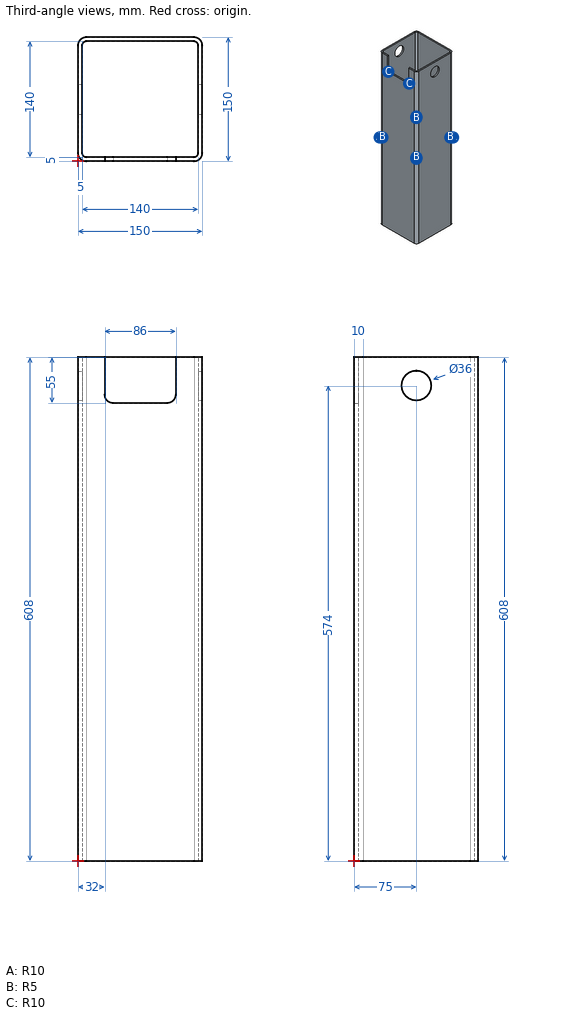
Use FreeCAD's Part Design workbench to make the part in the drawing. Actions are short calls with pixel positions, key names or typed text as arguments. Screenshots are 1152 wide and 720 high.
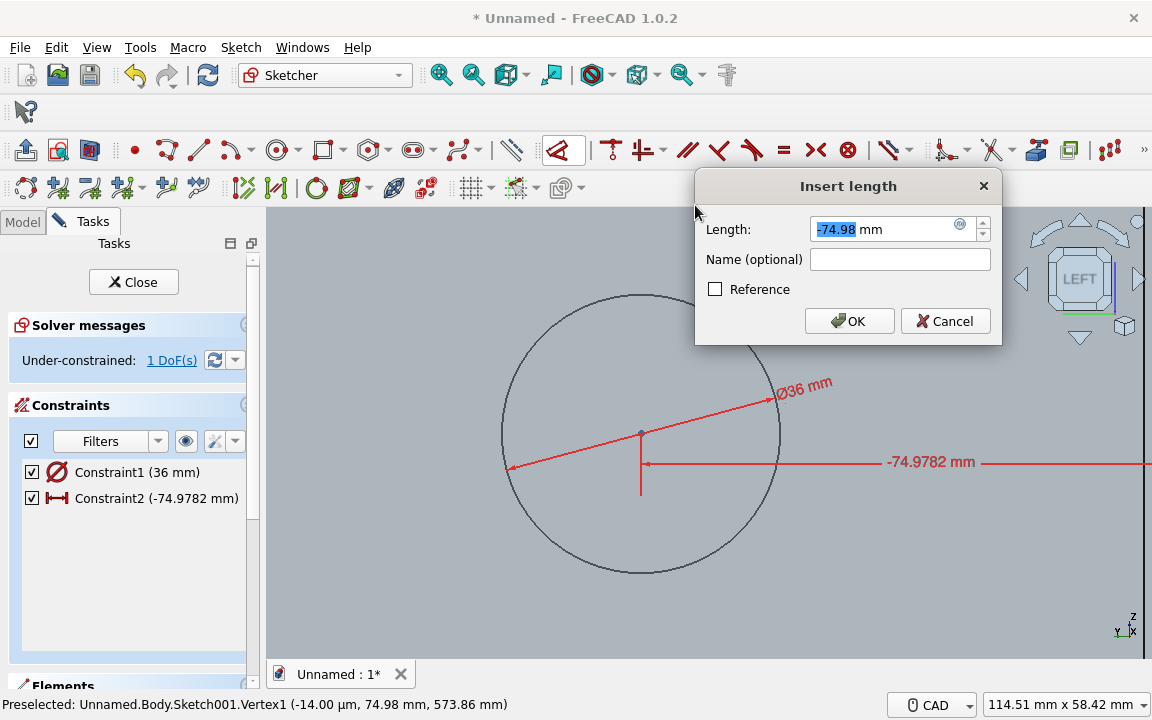
text(-75)
key(Return)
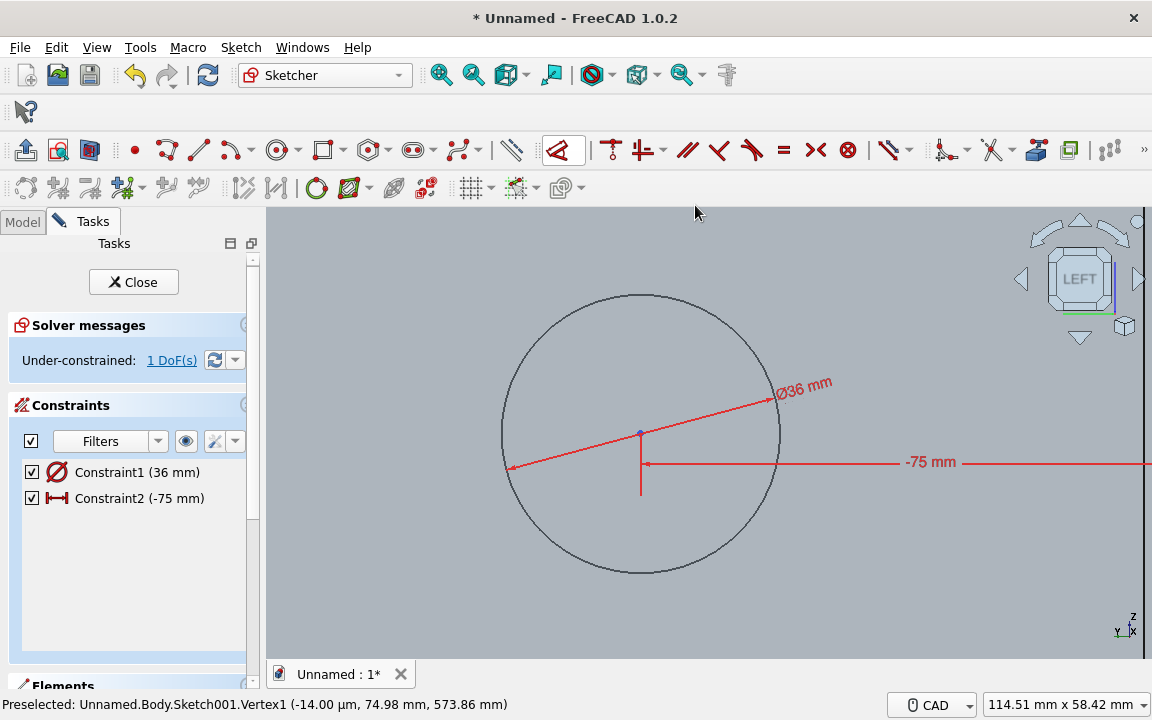
click(641, 434)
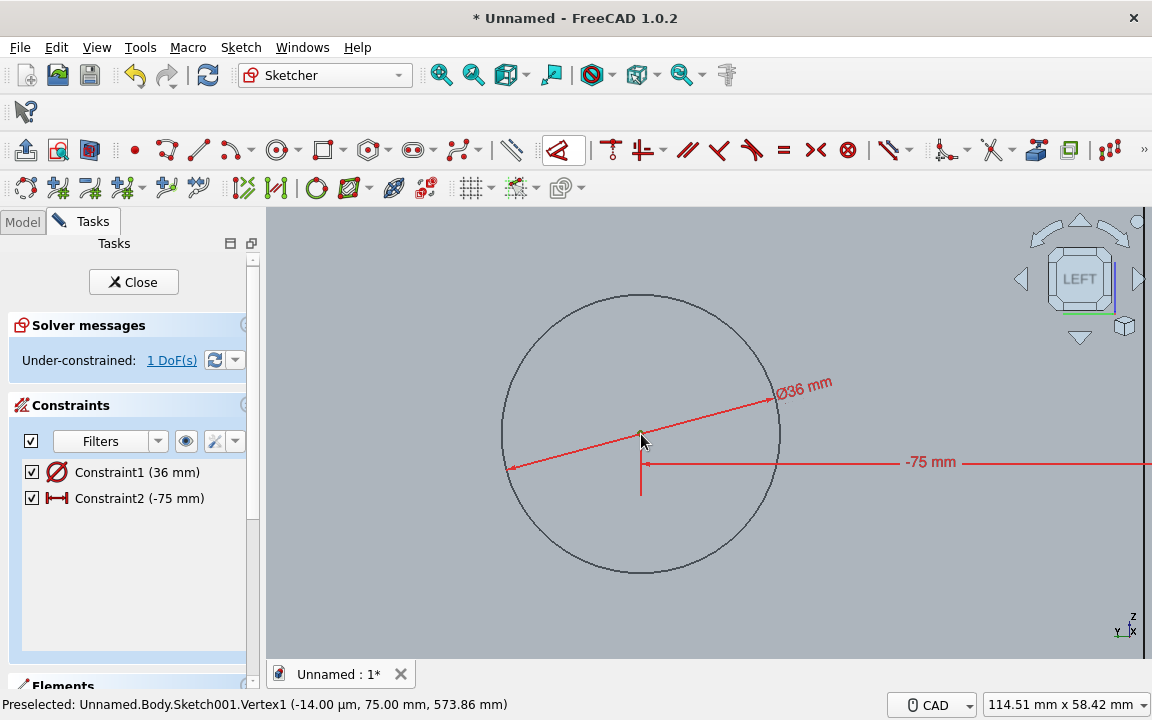
key(i)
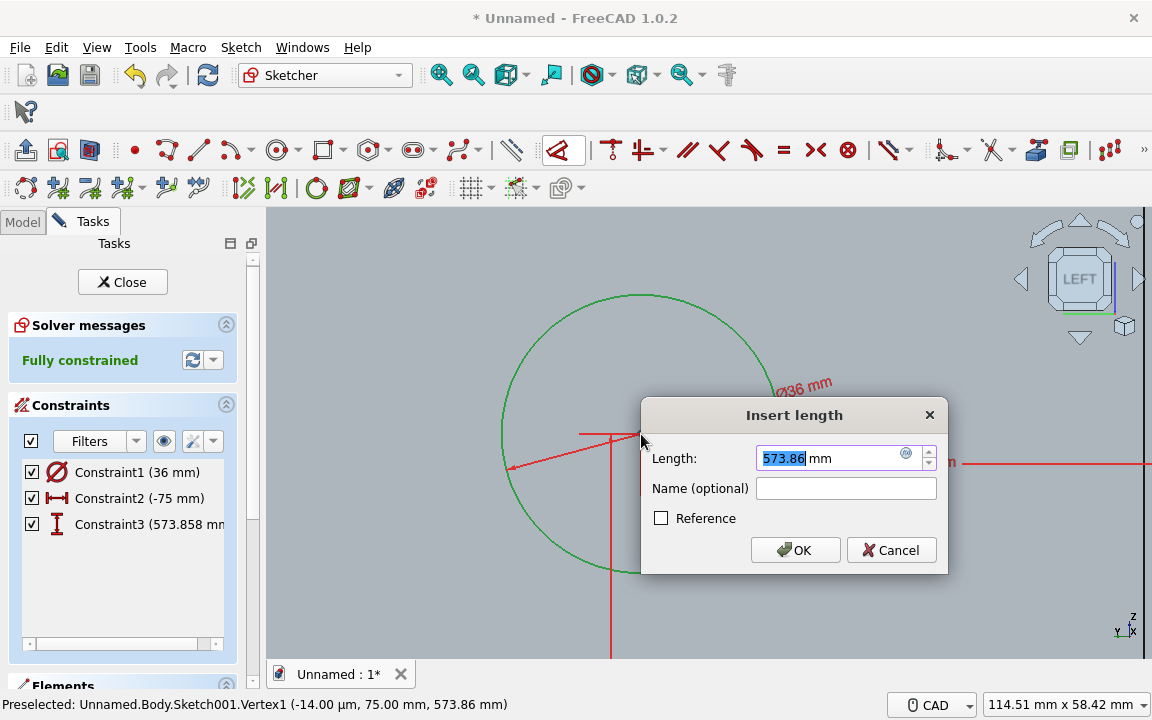
text(574)
key(Return)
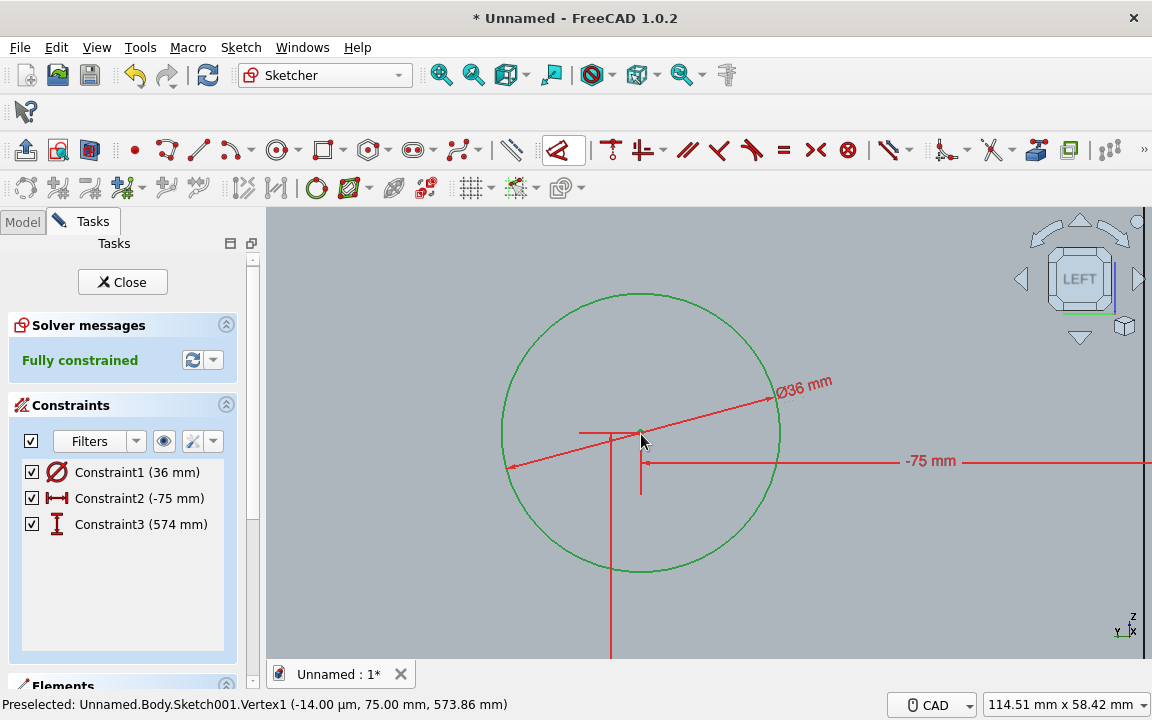
click(123, 282)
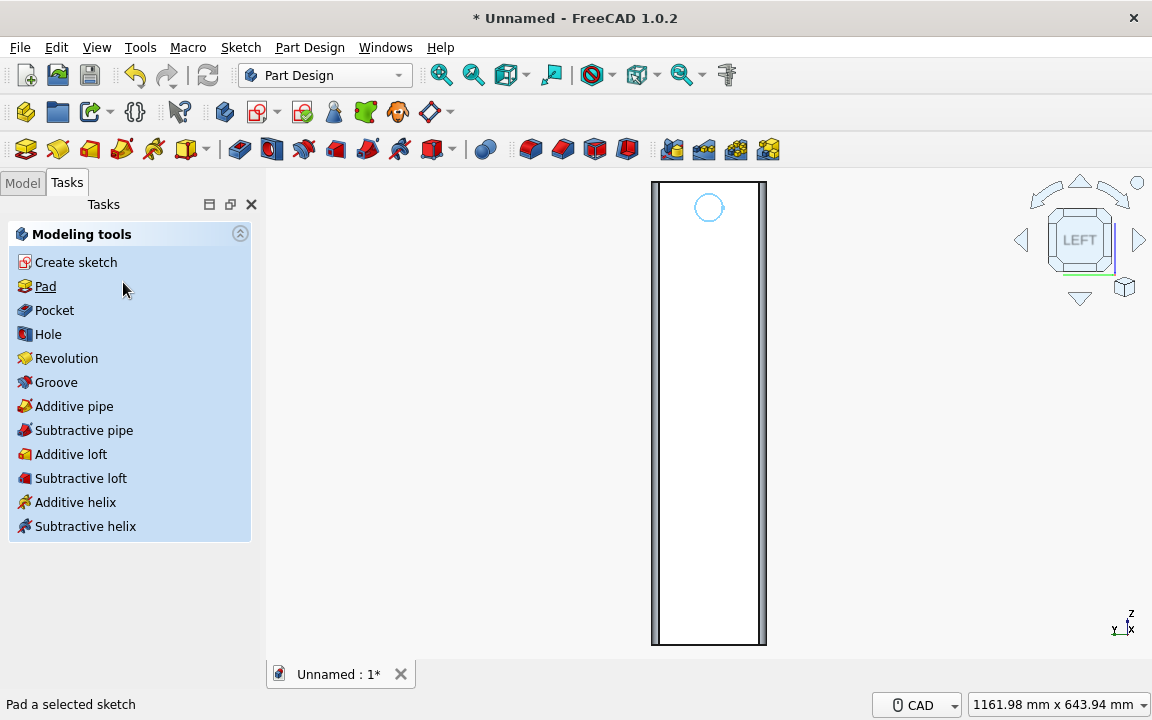
click(240, 150)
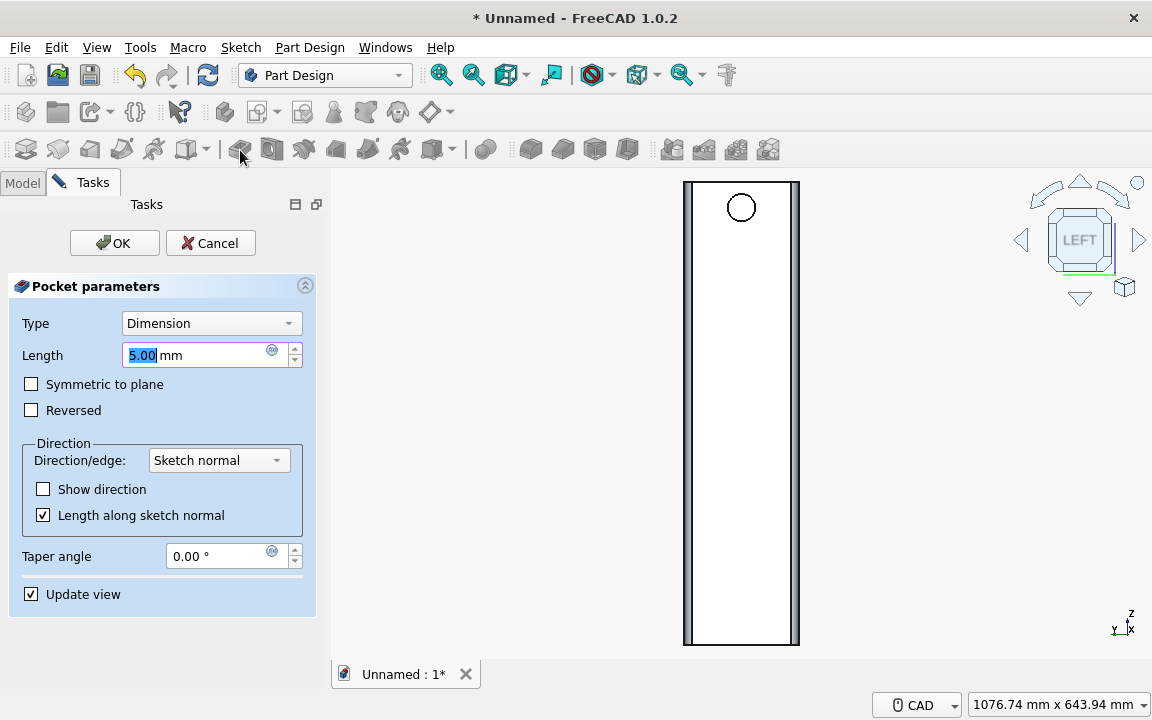
click(212, 324)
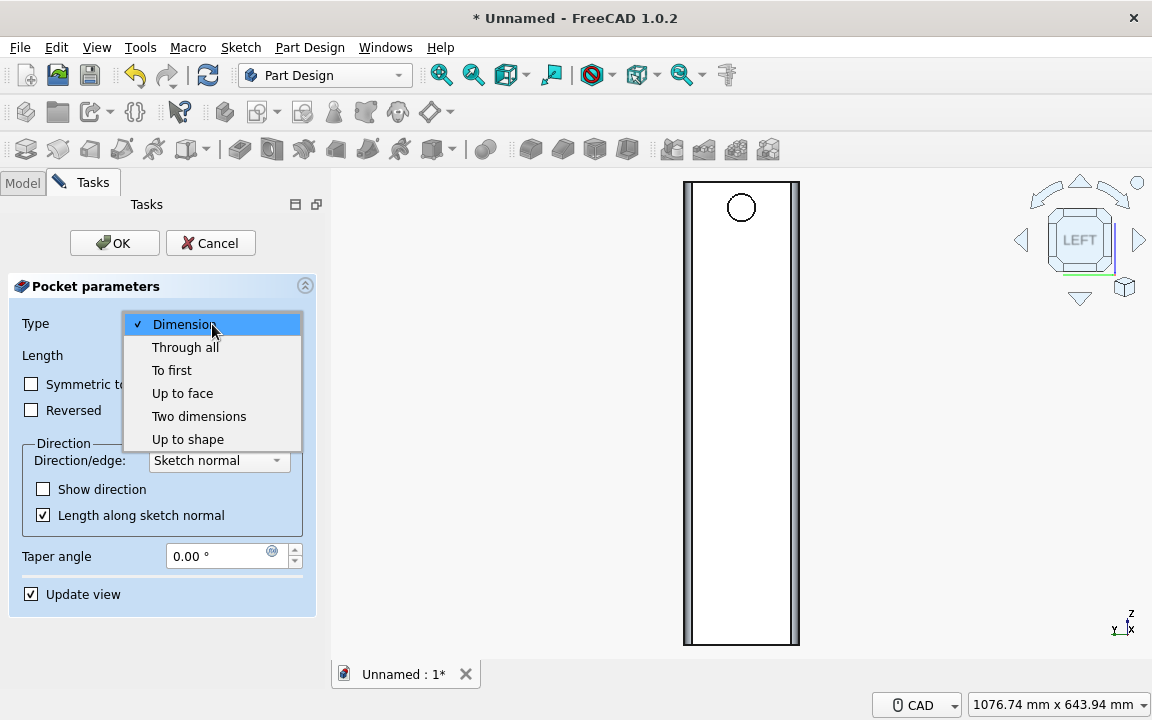
click(212, 348)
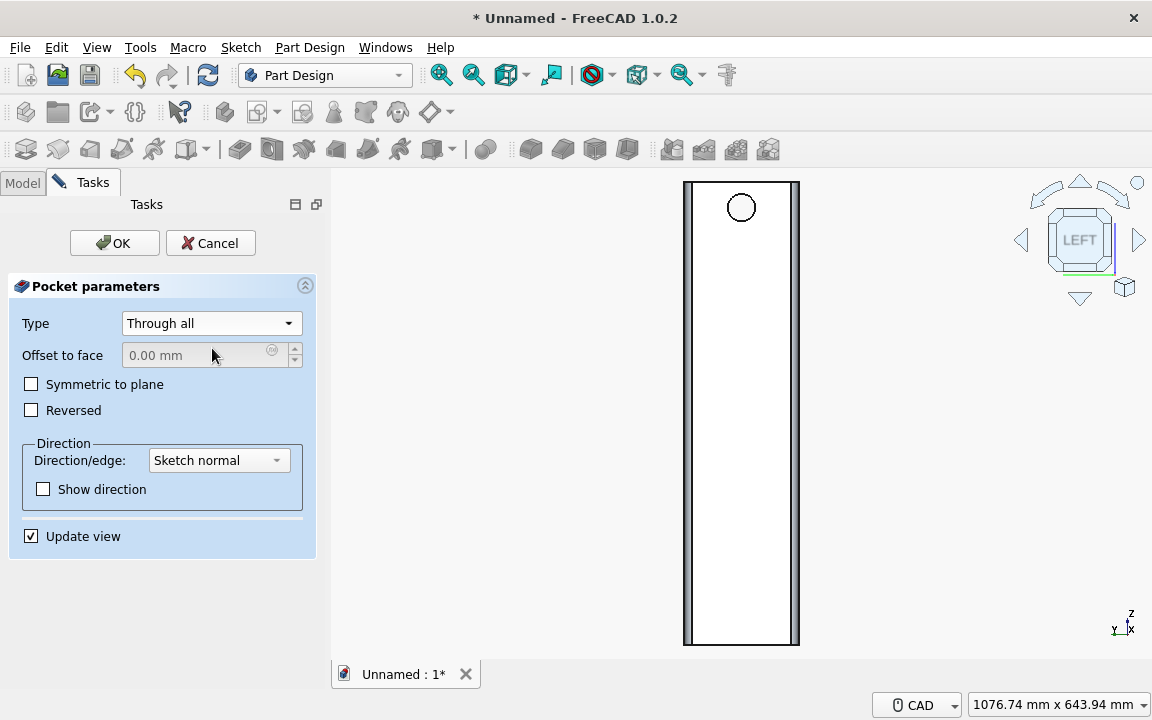
click(115, 243)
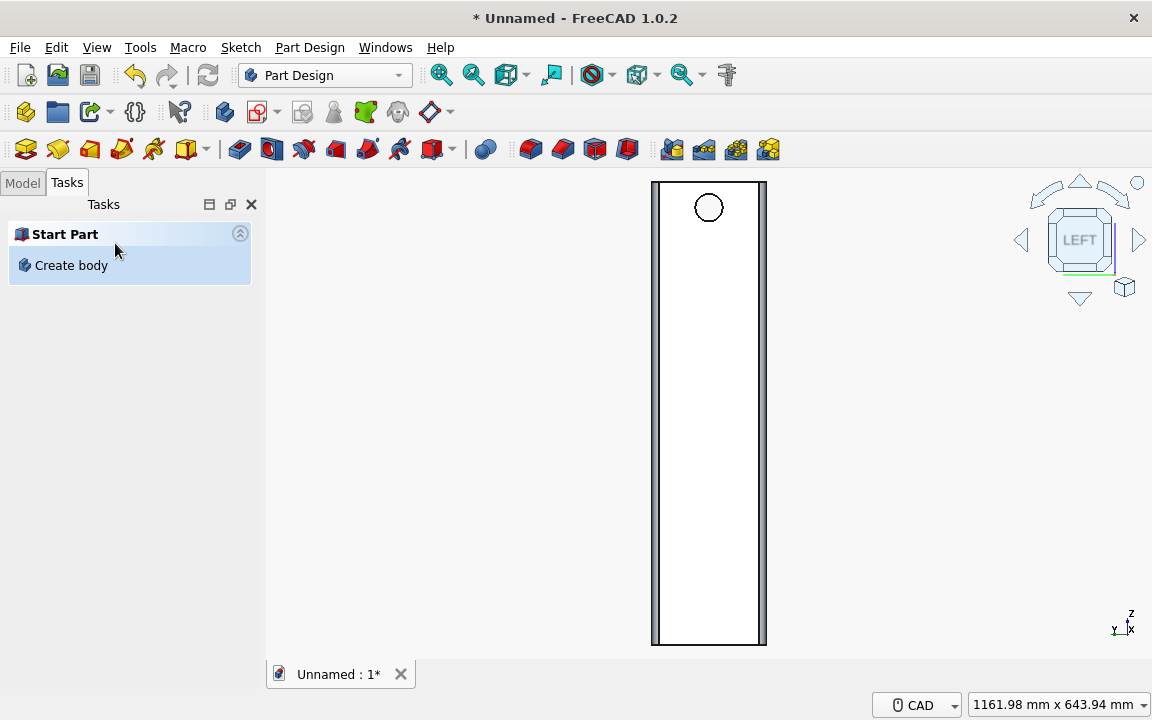
key(0)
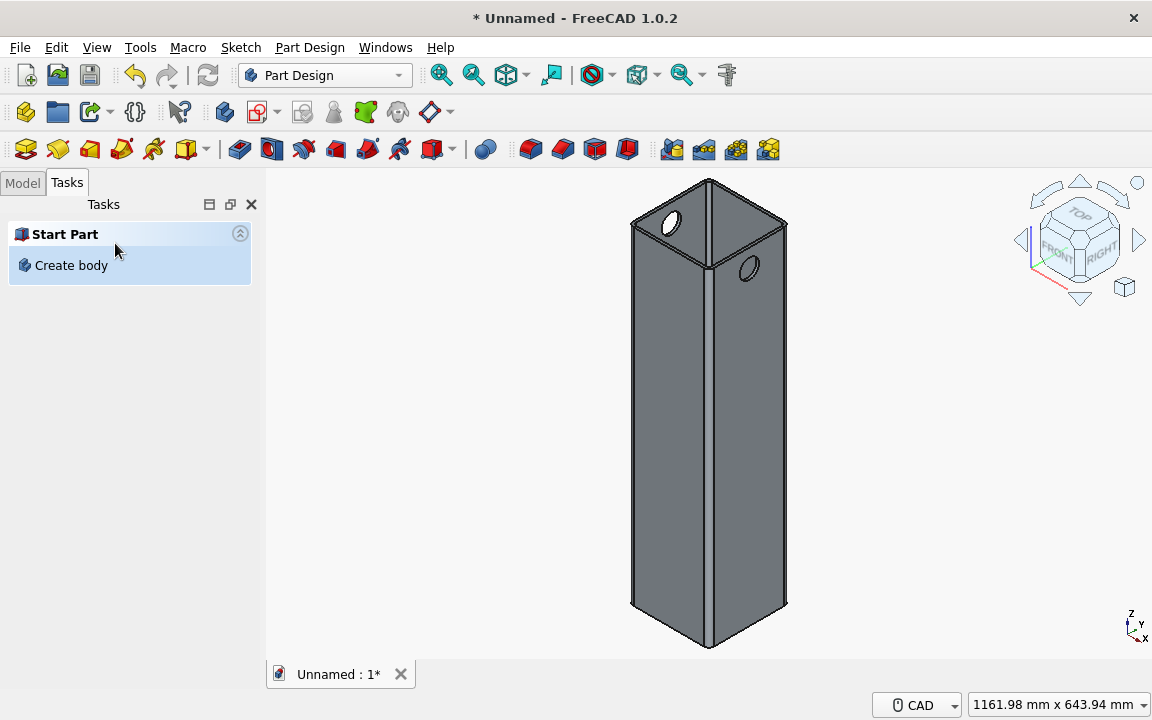
click(669, 328)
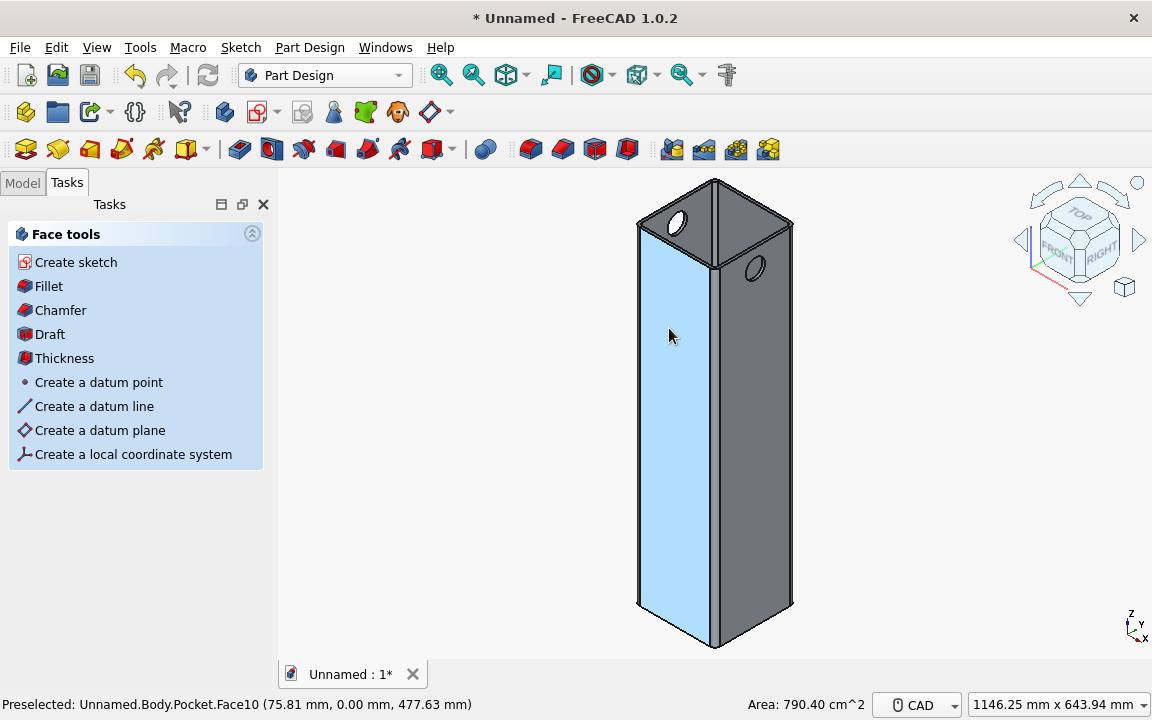
click(258, 112)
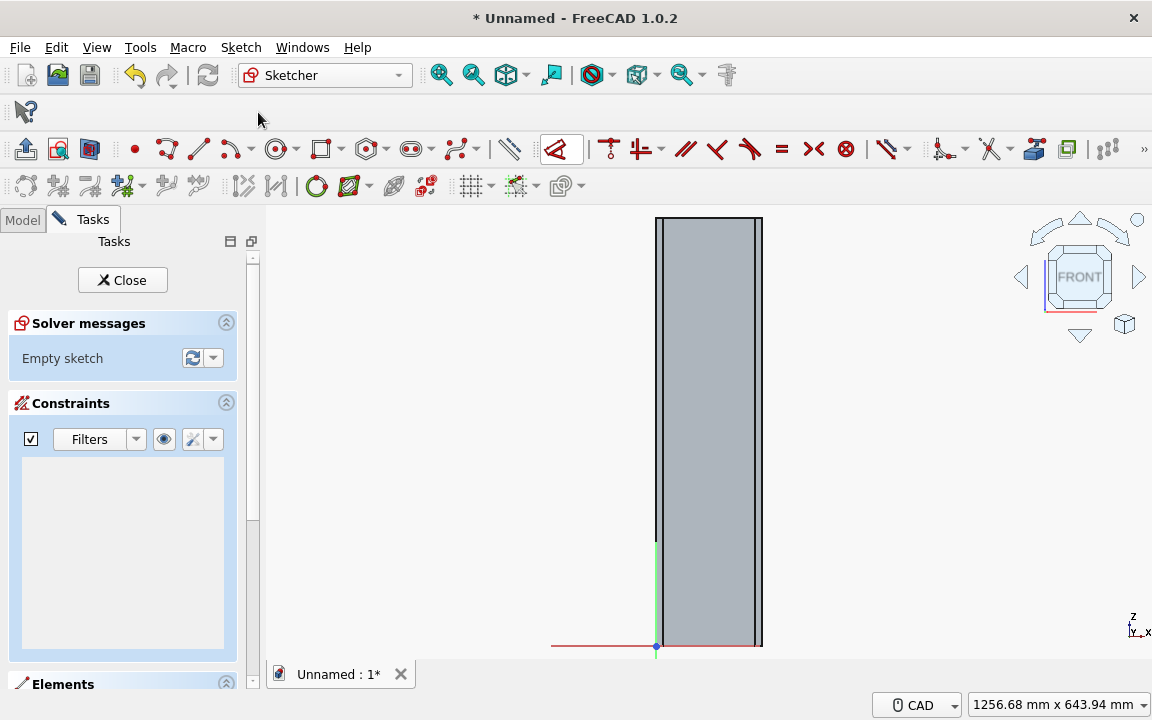
scroll(640, 432, down, 5)